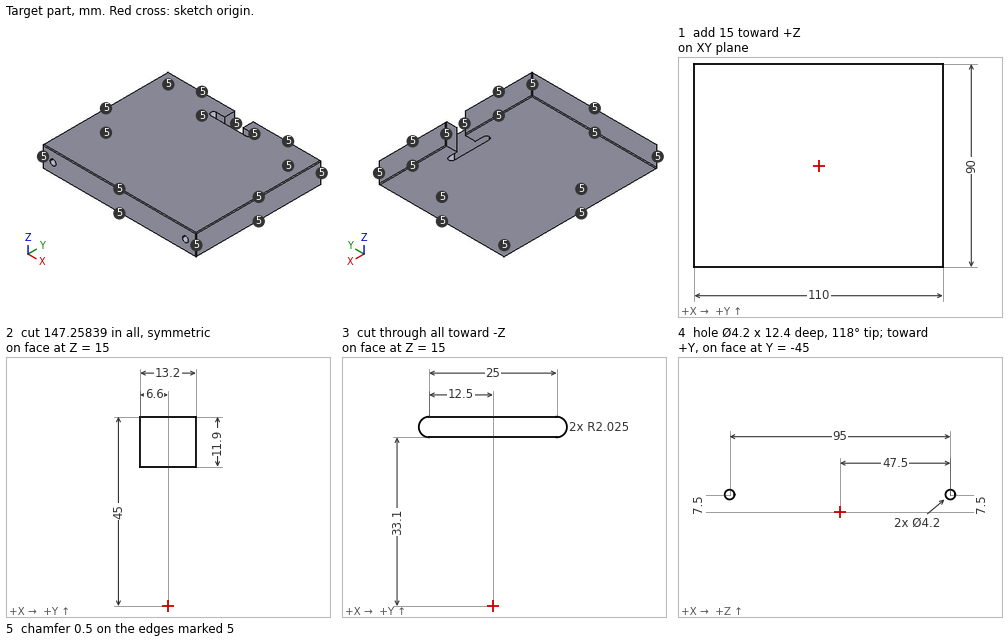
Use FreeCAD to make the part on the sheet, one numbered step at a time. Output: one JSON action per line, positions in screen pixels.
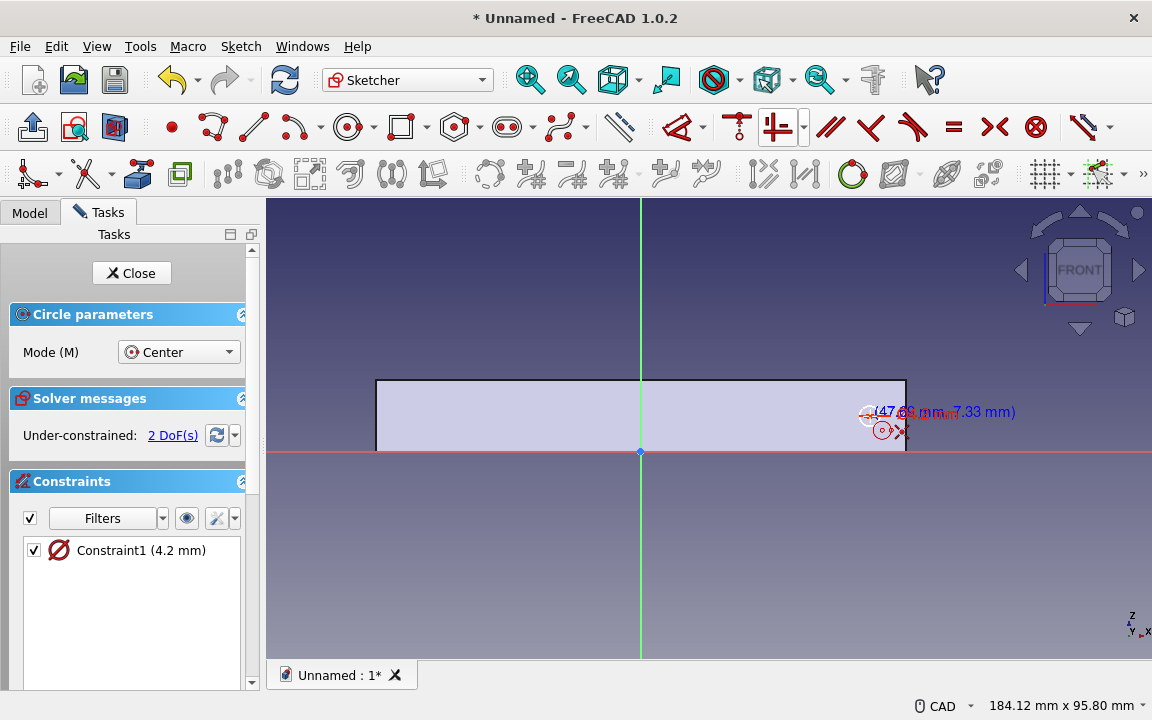
{"action": "scroll", "coordinate": [412, 416], "scroll_direction": "up", "scroll_amount": 5}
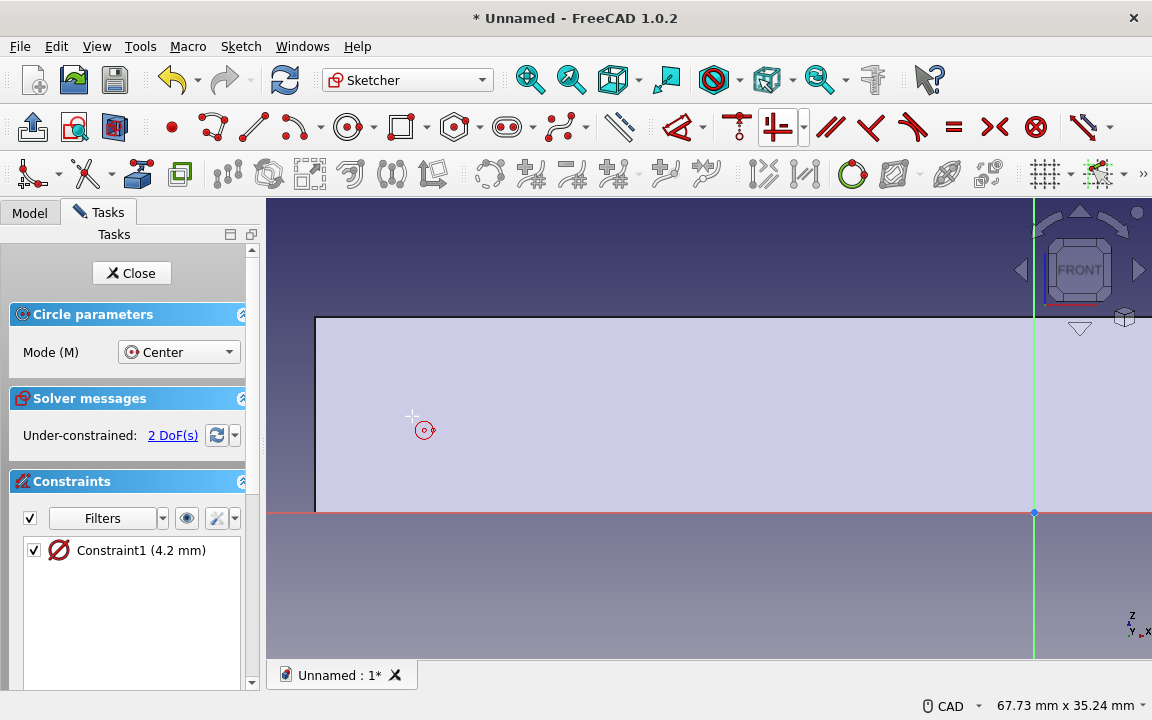
{"action": "left_click", "coordinate": [413, 415]}
{"action": "mouse_move", "coordinate": [432, 395]}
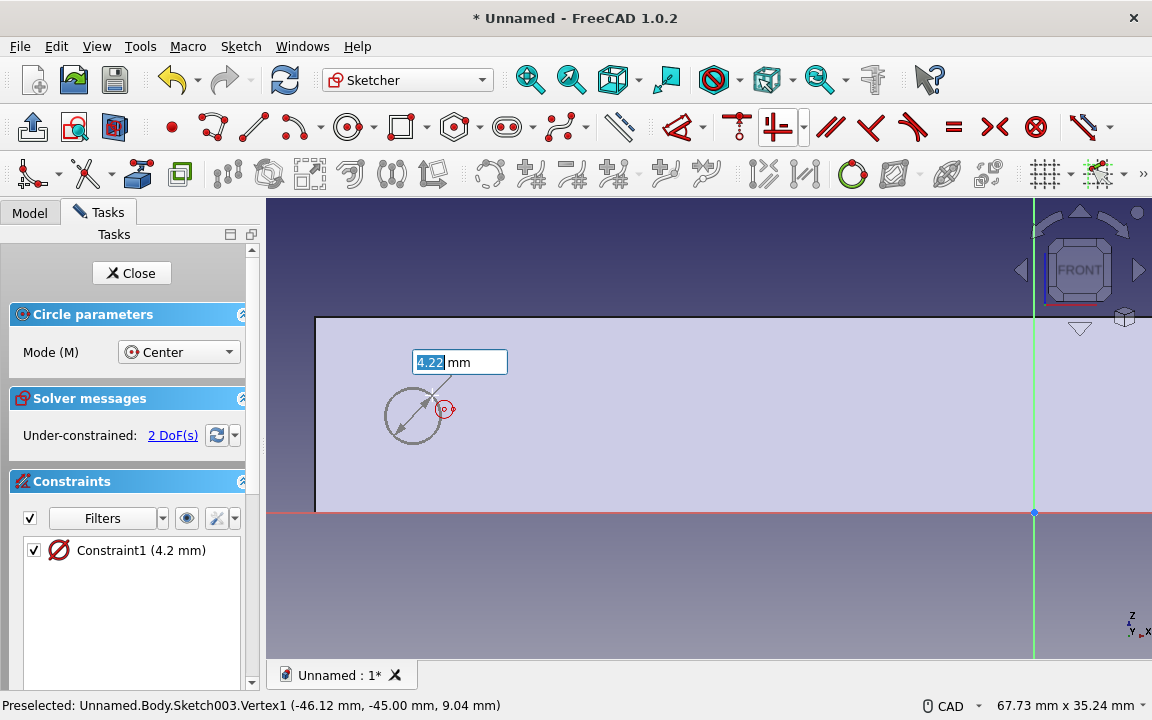
{"action": "type", "text": "4.2"}
{"action": "key", "text": "Return"}
{"action": "key", "text": "Escape"}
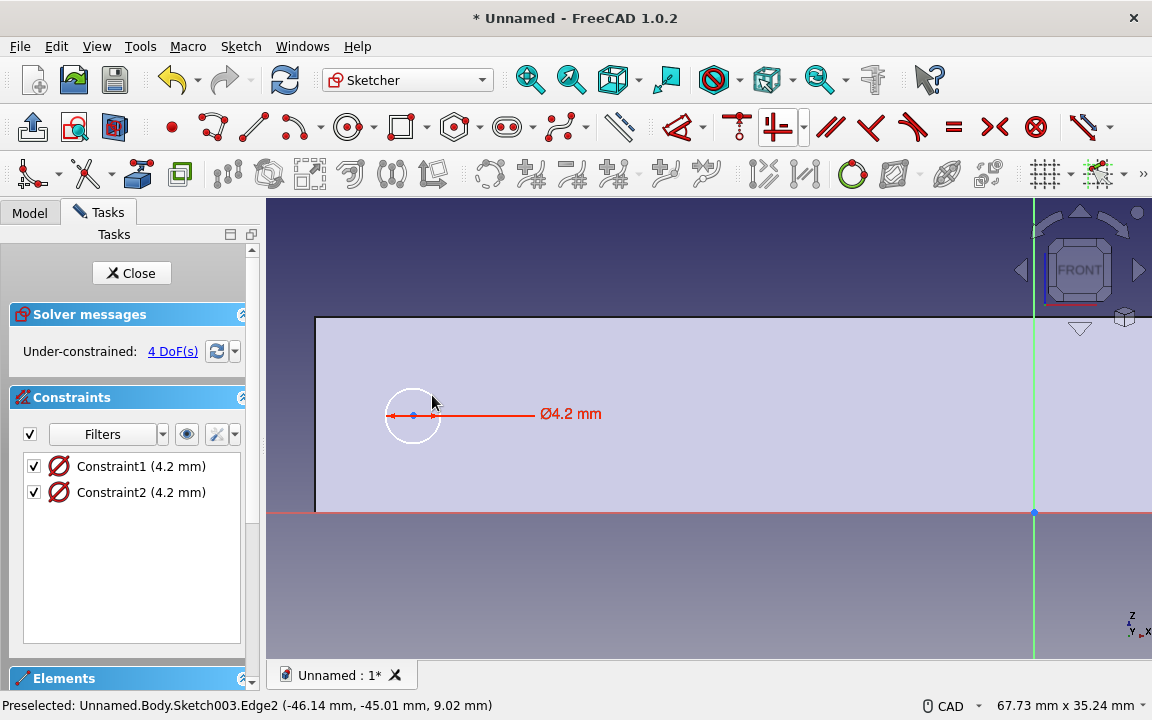
{"action": "left_click", "coordinate": [676, 128]}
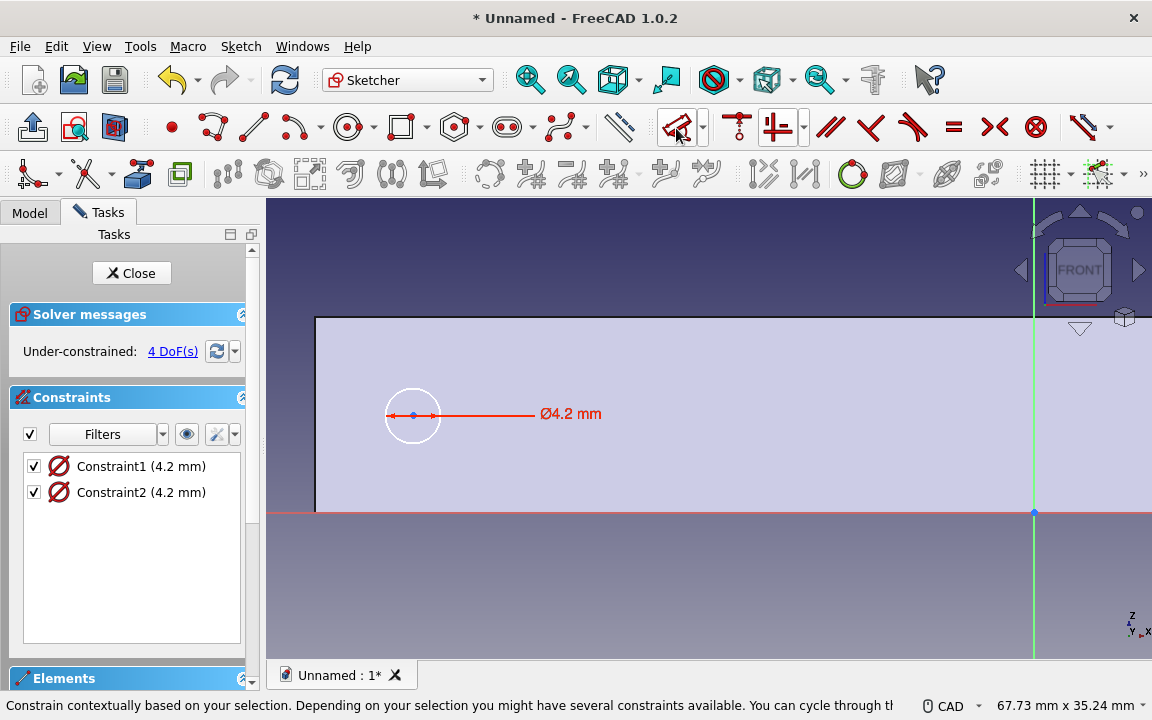
{"action": "scroll", "coordinate": [411, 416], "scroll_direction": "down", "scroll_amount": 5}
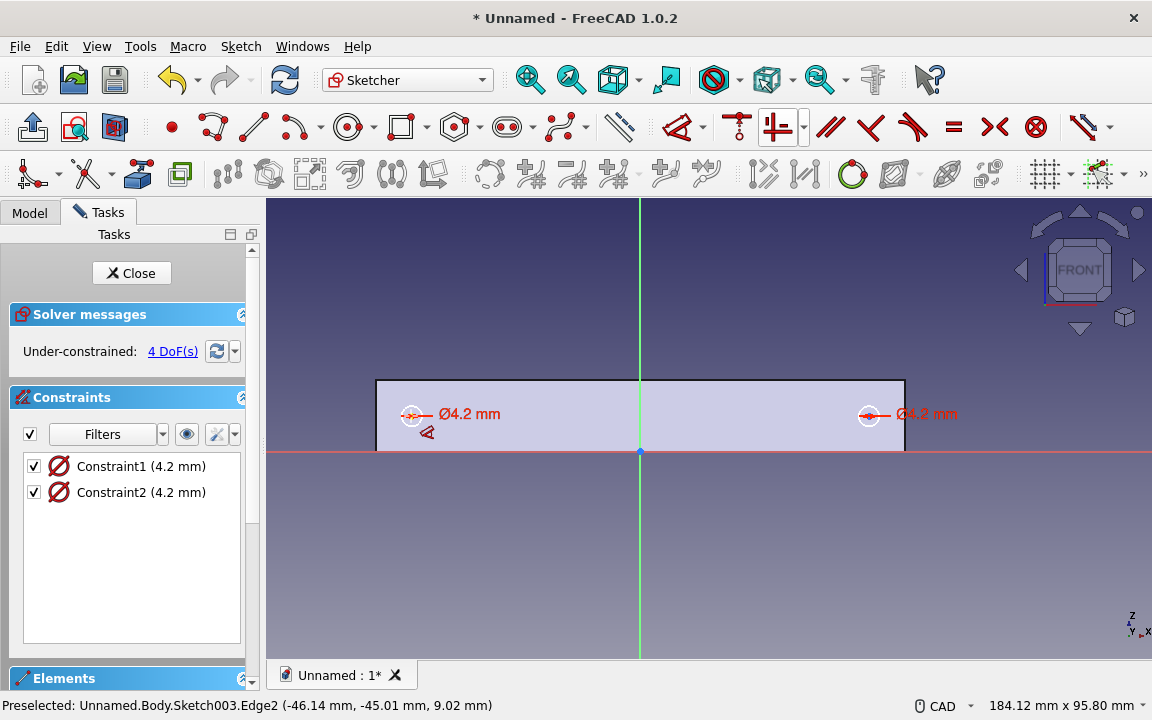
{"action": "left_click", "coordinate": [869, 416]}
{"action": "left_click", "coordinate": [903, 434]}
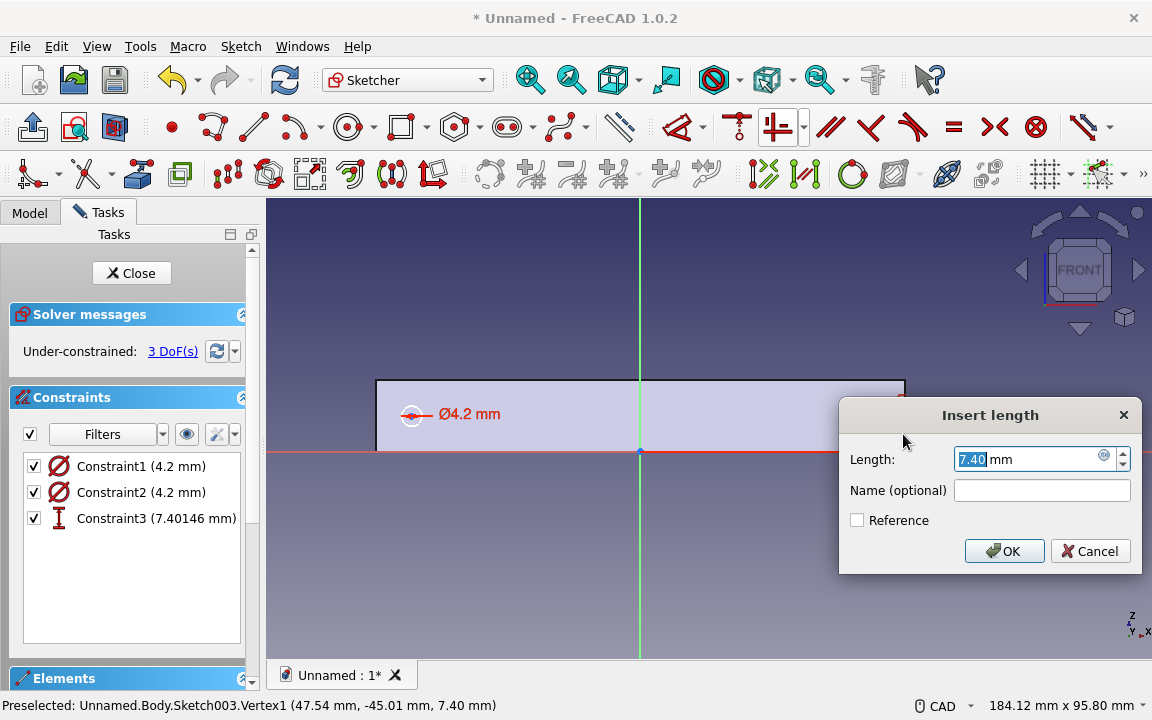
{"action": "type", "text": "7.5"}
{"action": "key", "text": "Return"}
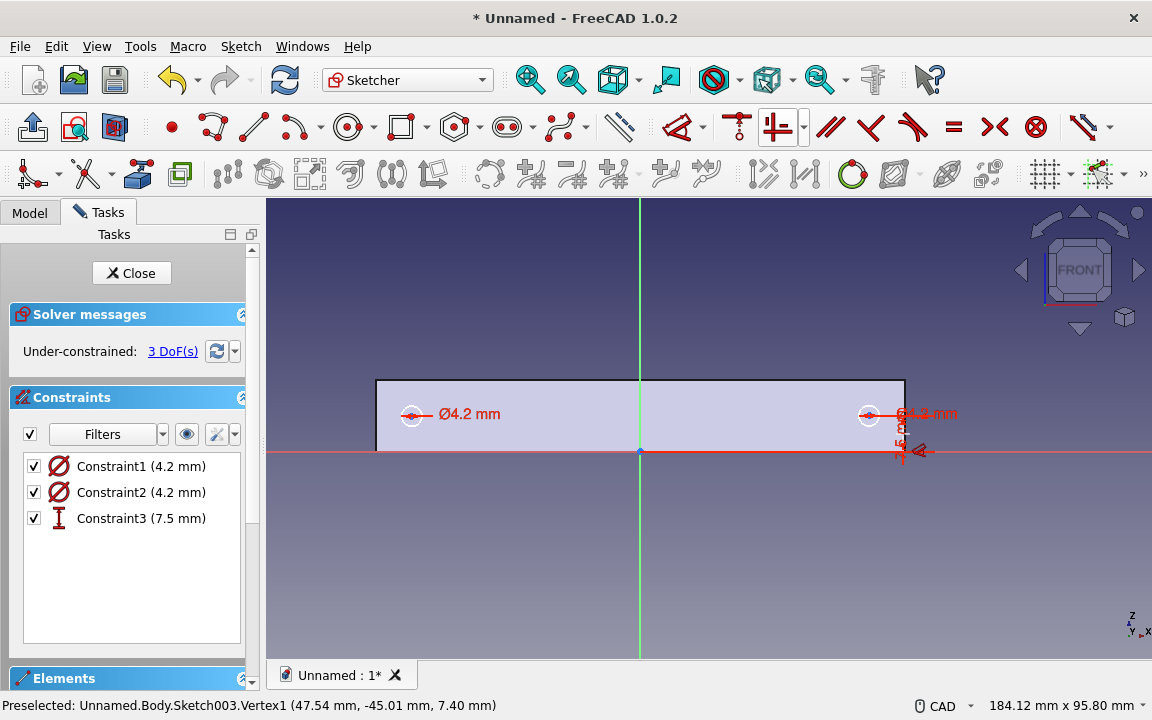
{"action": "left_click", "coordinate": [412, 416]}
{"action": "left_click", "coordinate": [378, 434]}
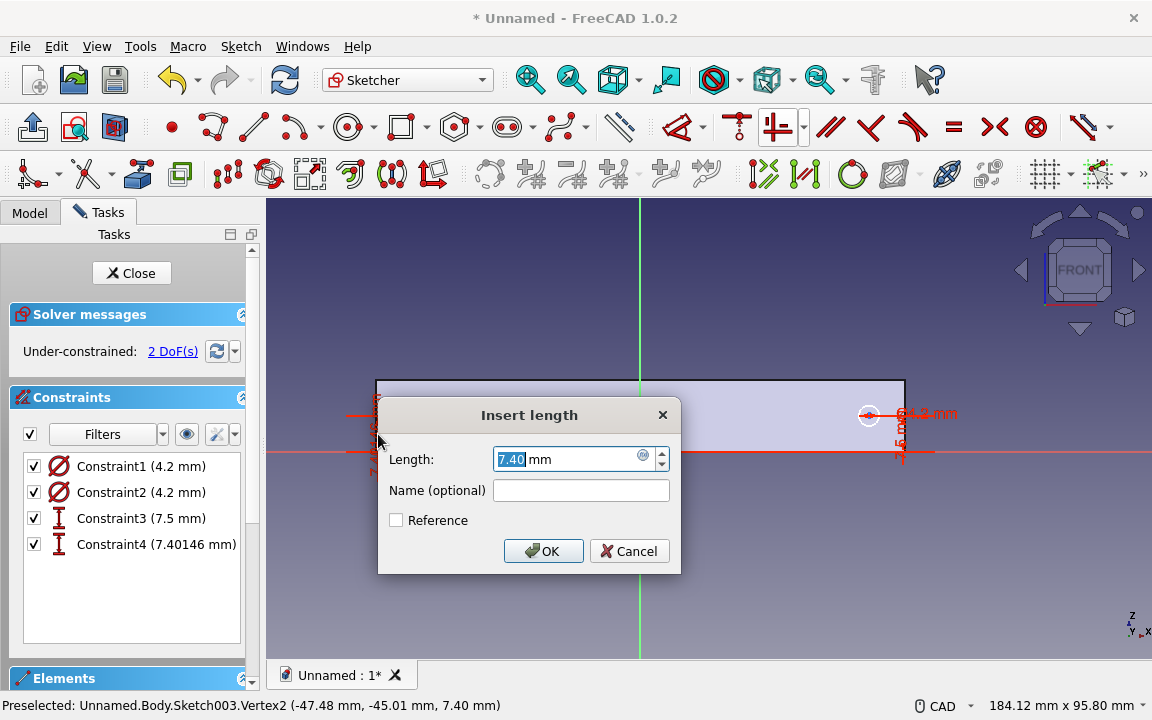
{"action": "type", "text": "7.5"}
{"action": "key", "text": "Return"}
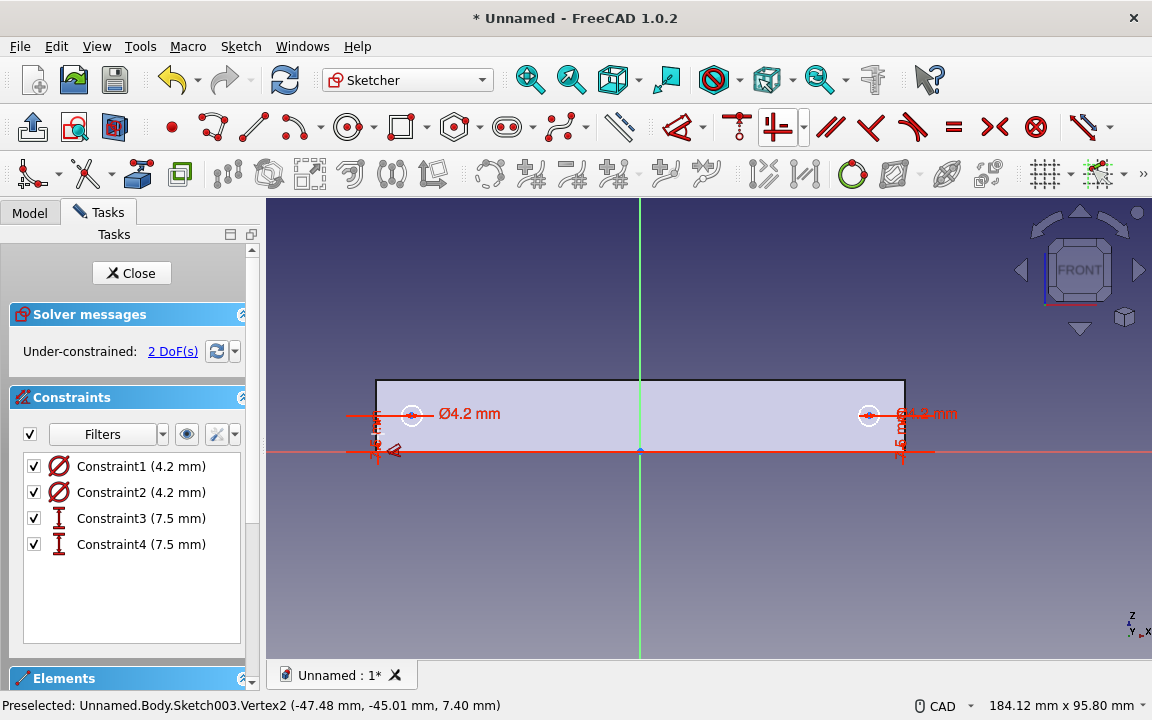
{"action": "left_click", "coordinate": [869, 416]}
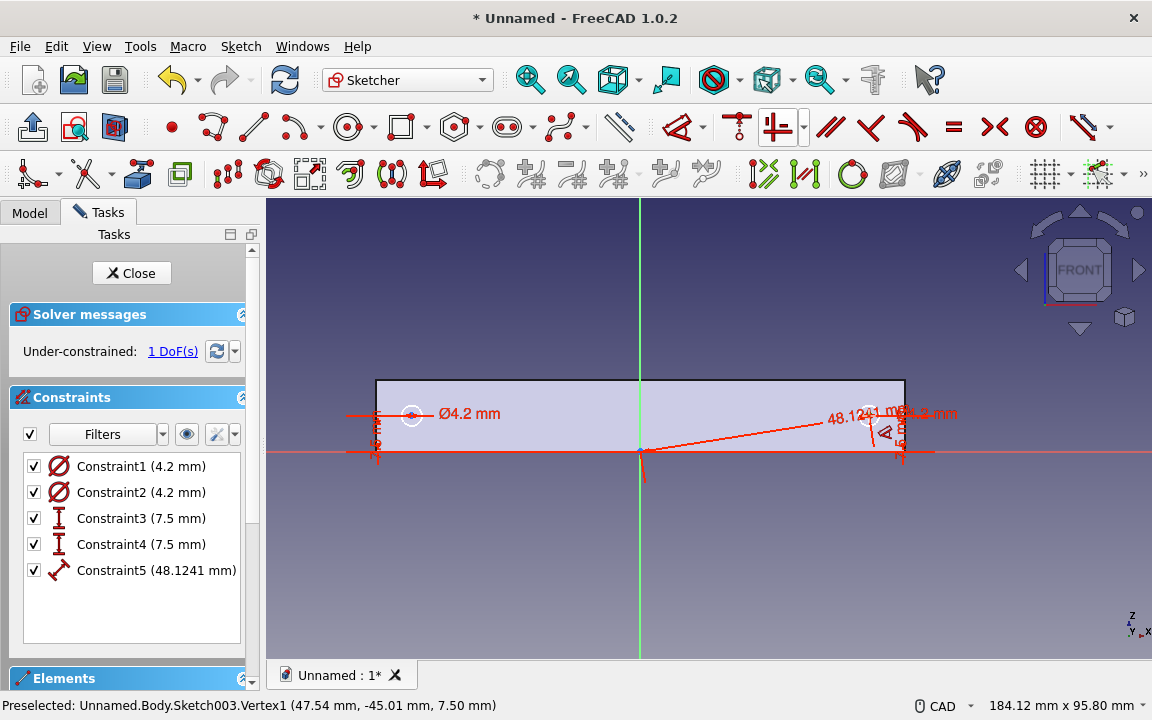
{"action": "left_click", "coordinate": [412, 416]}
{"action": "left_click", "coordinate": [535, 382]}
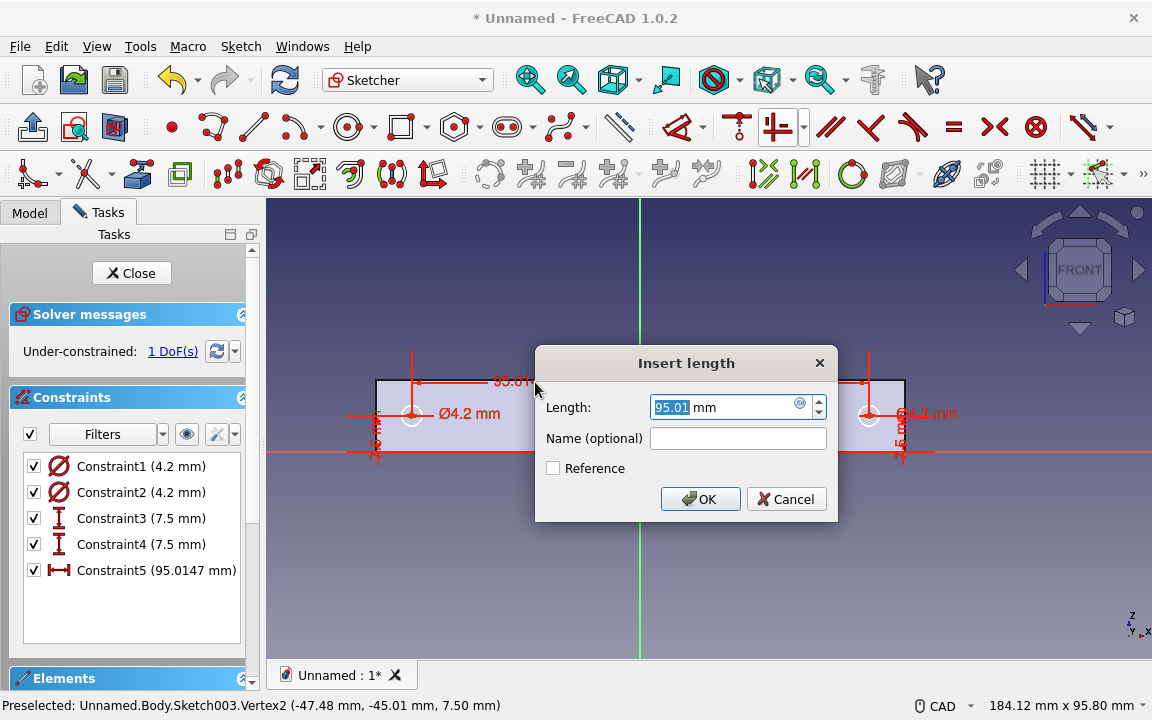
{"action": "type", "text": "95"}
{"action": "key", "text": "Return"}